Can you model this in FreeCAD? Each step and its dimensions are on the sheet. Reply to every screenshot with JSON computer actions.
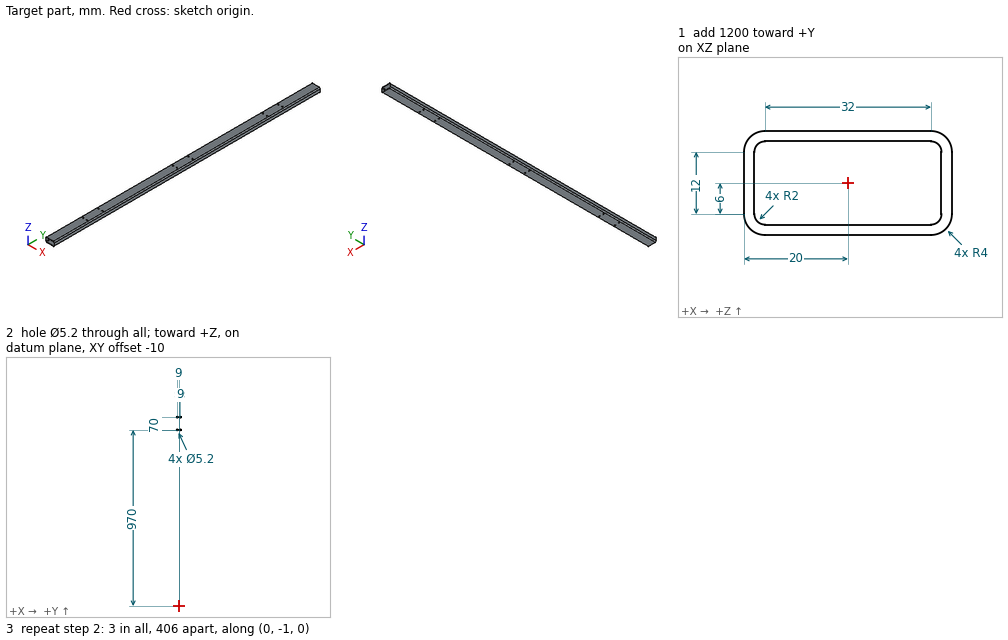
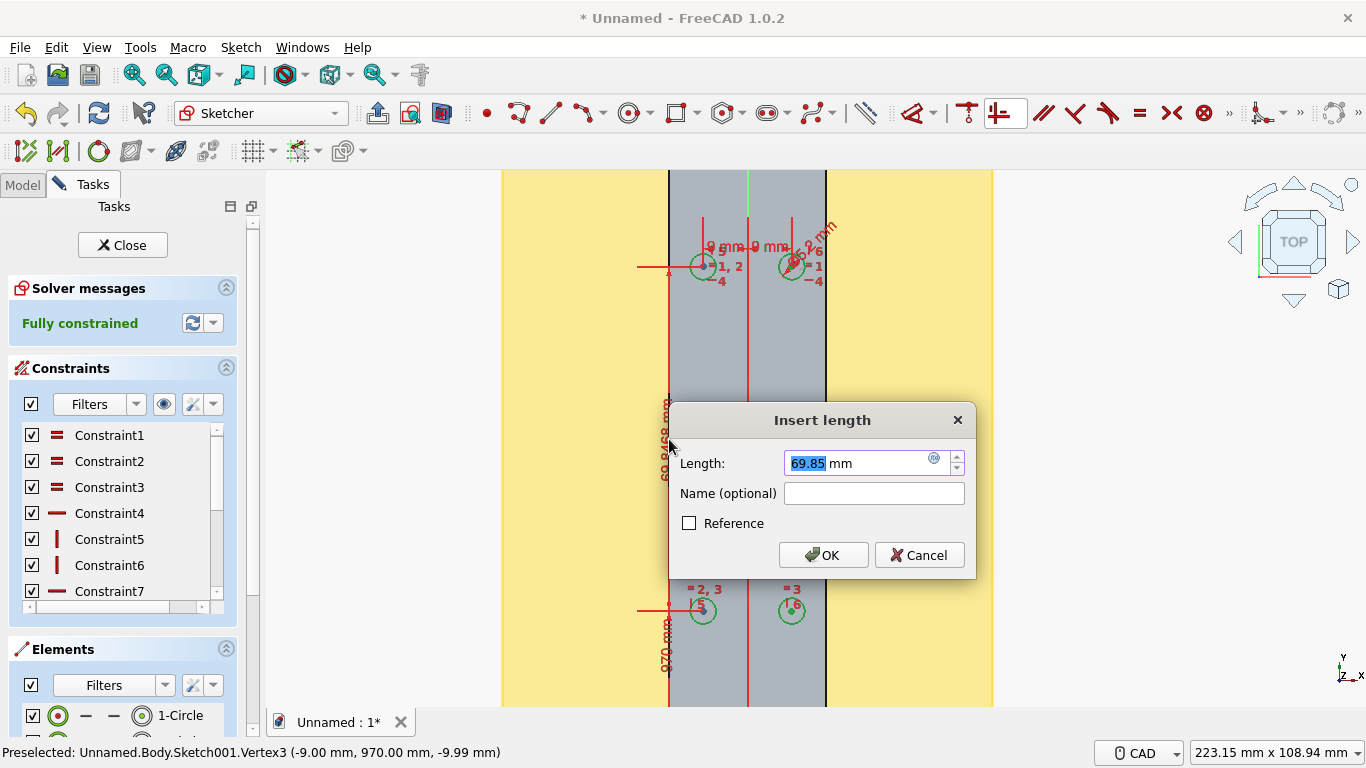
{"action": "type", "text": "70"}
{"action": "key", "text": "Return"}
{"action": "key", "text": "Escape"}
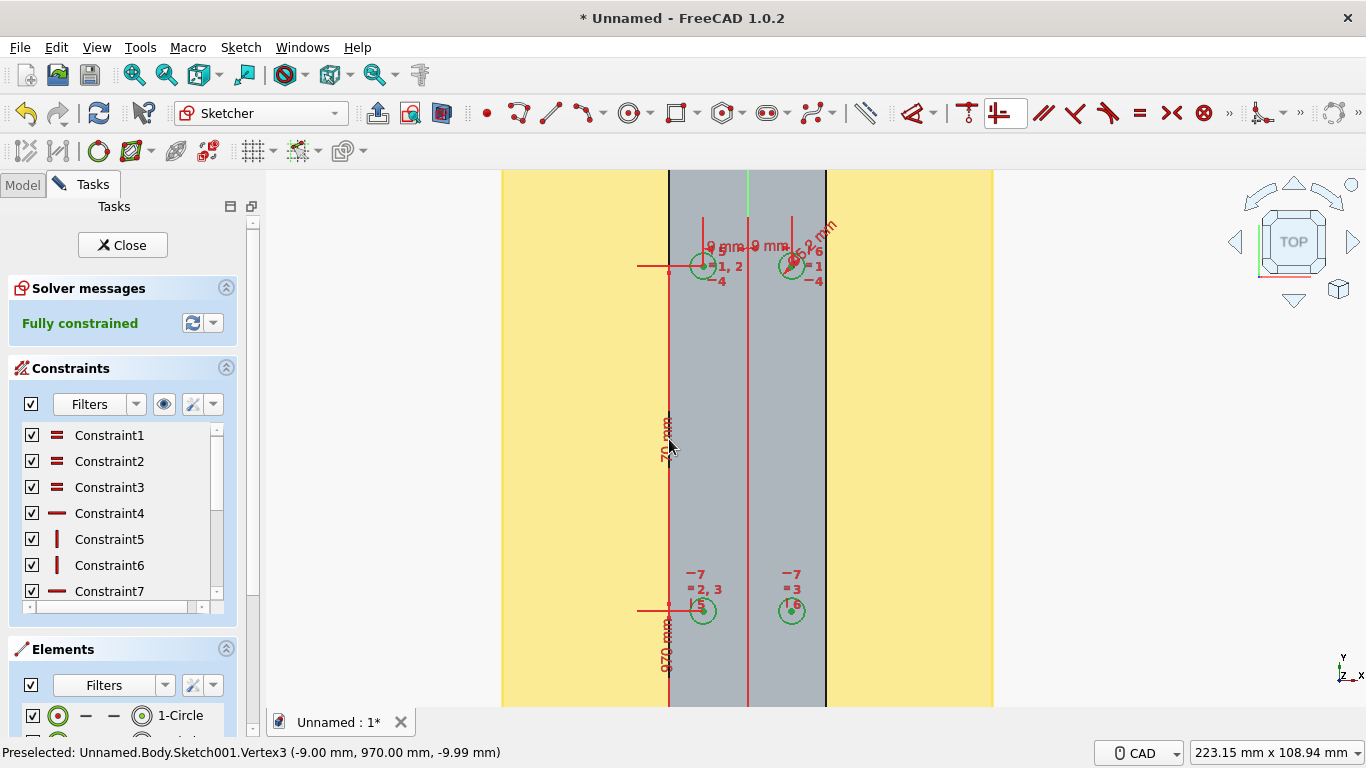
{"action": "left_click", "coordinate": [123, 245]}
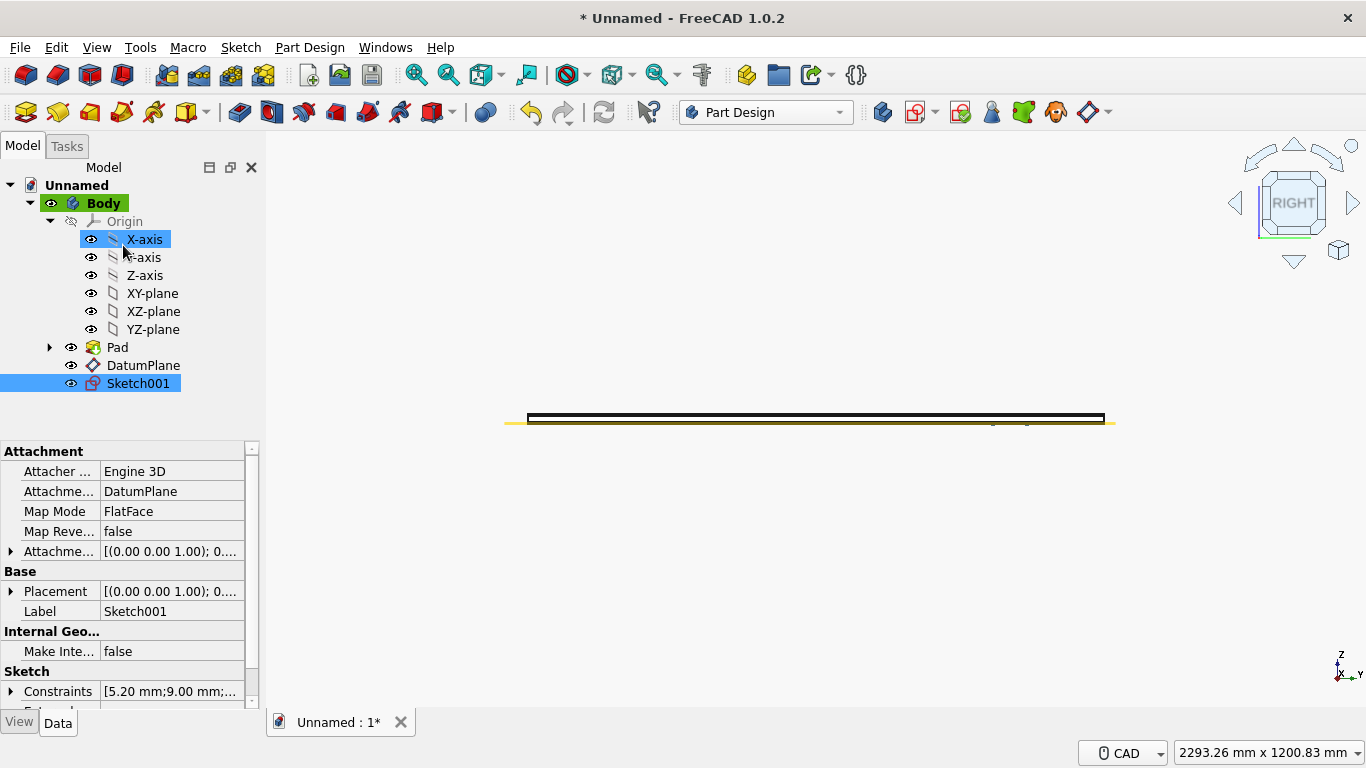
{"action": "left_click", "coordinate": [272, 112]}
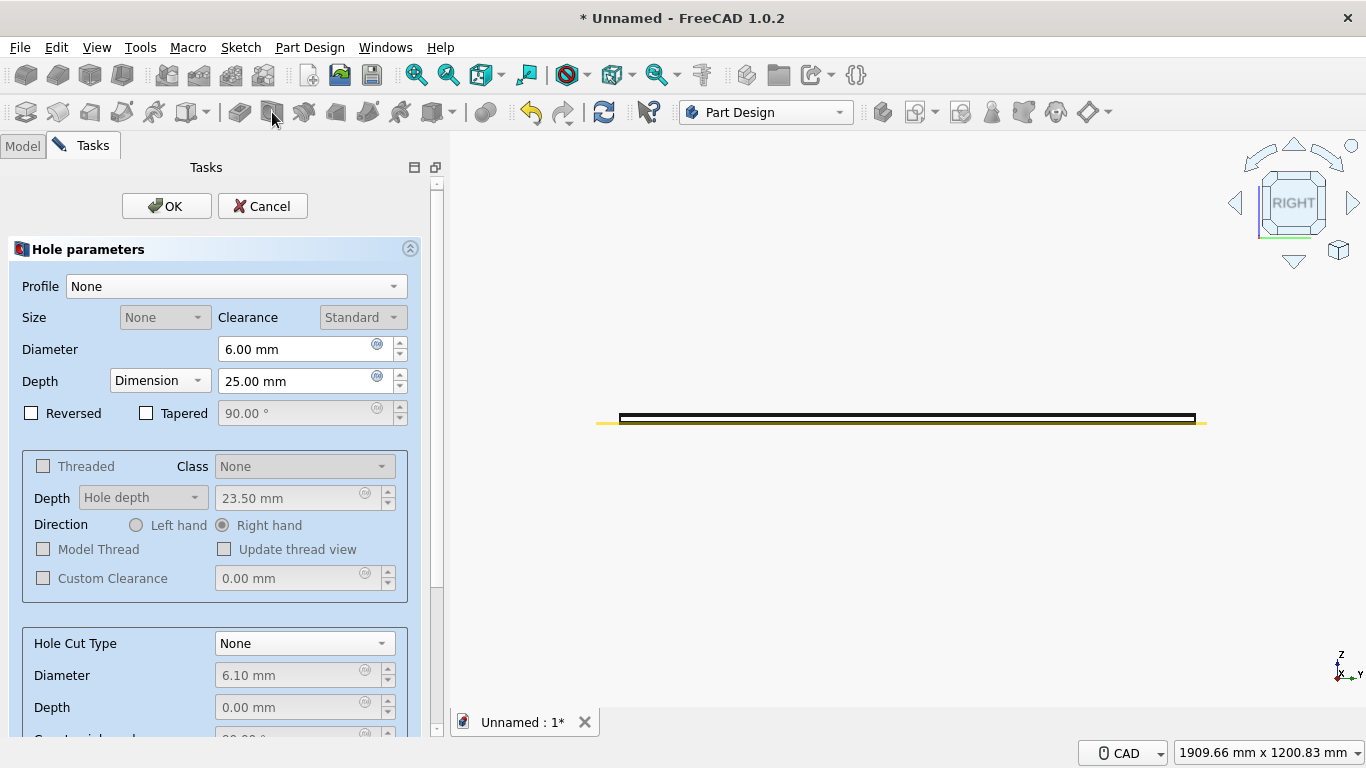
{"action": "triple_click", "coordinate": [305, 349]}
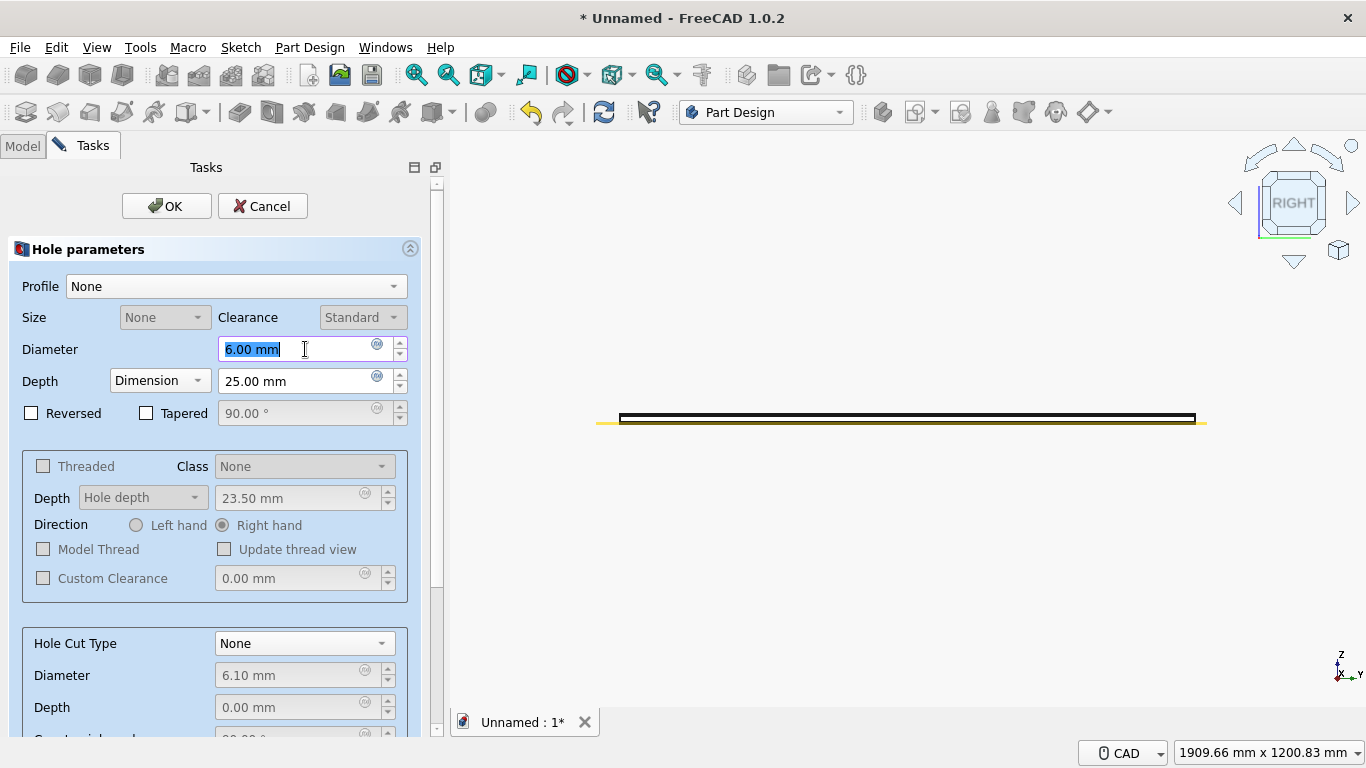
{"action": "type", "text": "5.2"}
{"action": "key", "text": "Tab"}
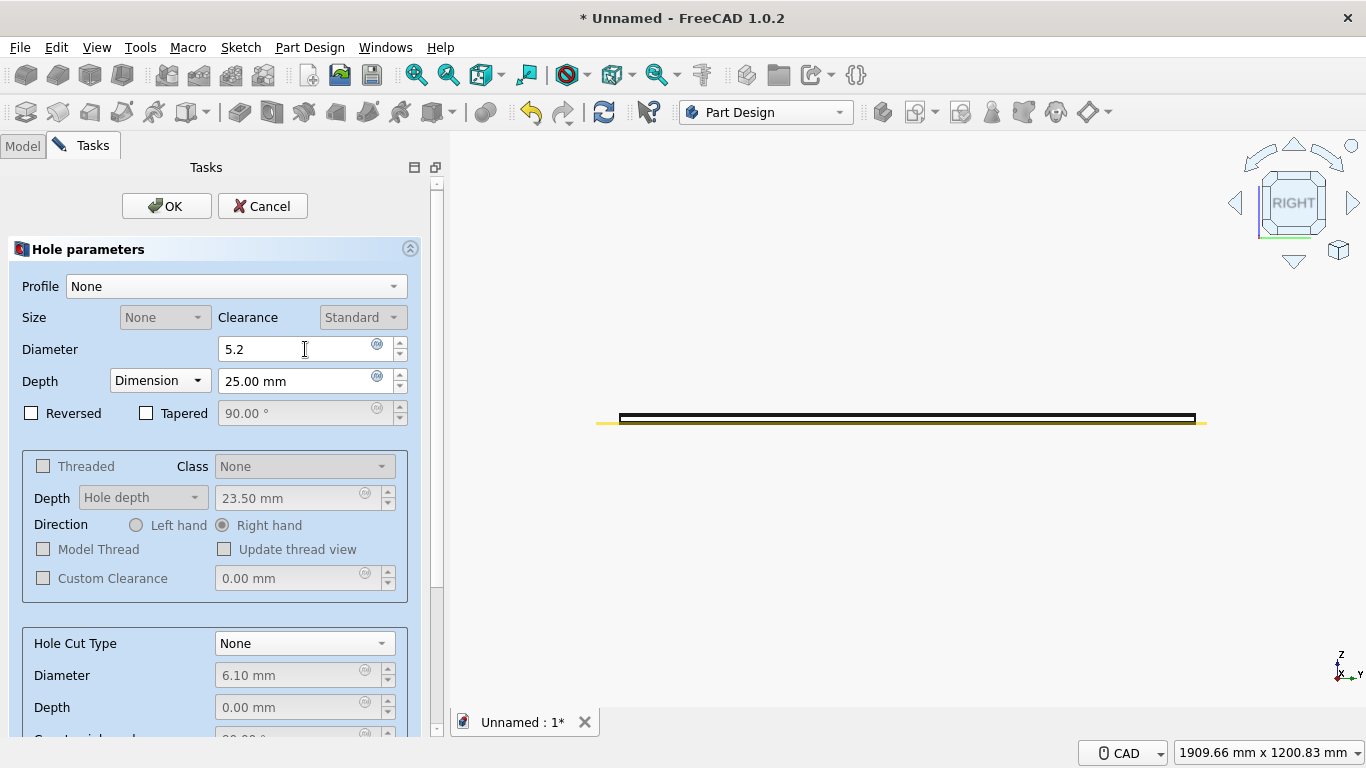
{"action": "left_click", "coordinate": [161, 380]}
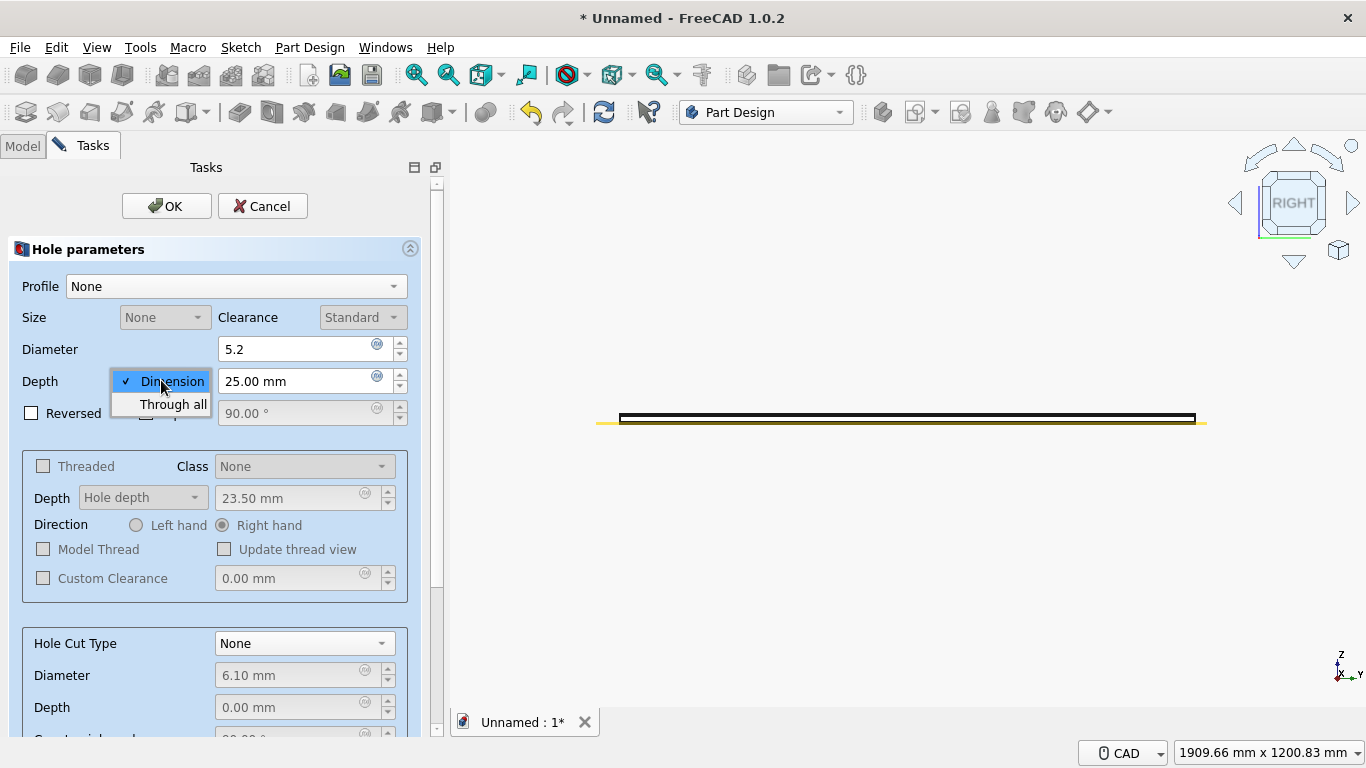
{"action": "left_click", "coordinate": [160, 404]}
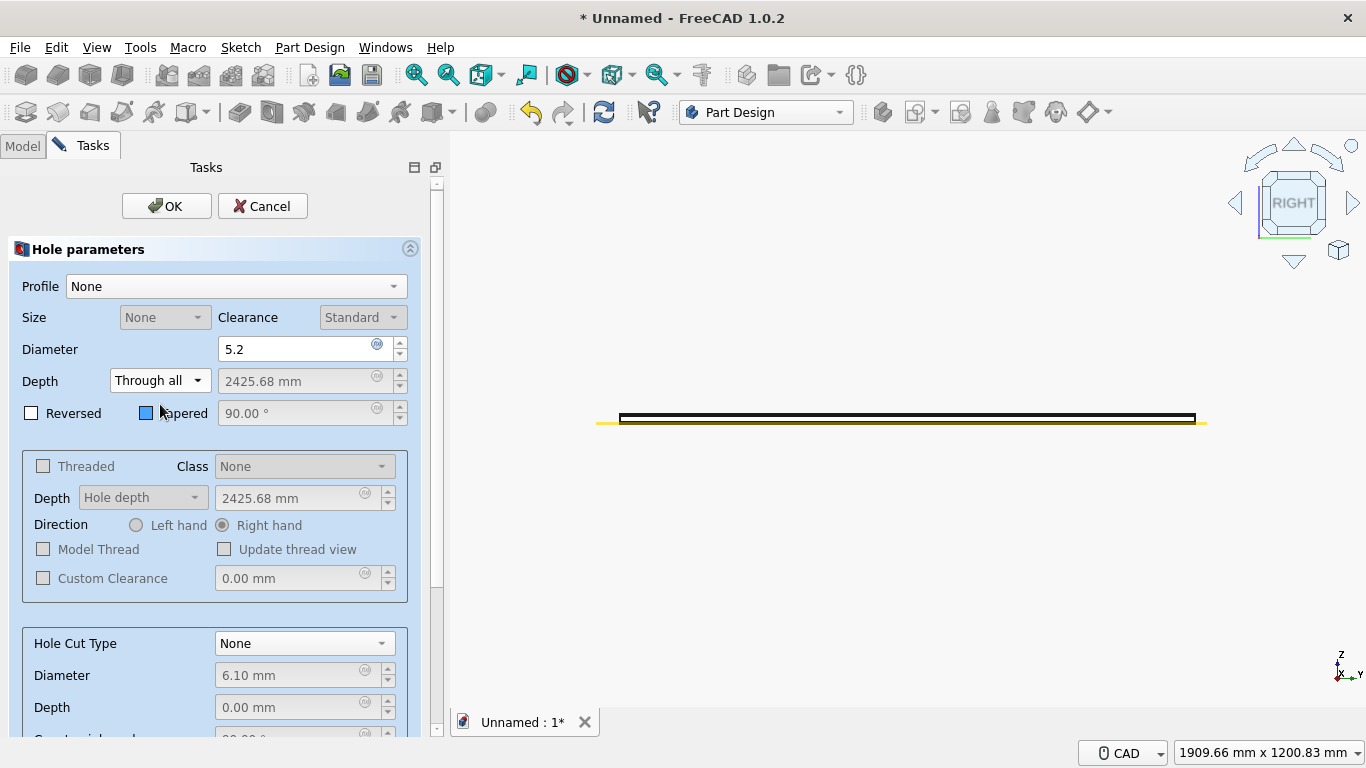
{"action": "left_click", "coordinate": [30, 413]}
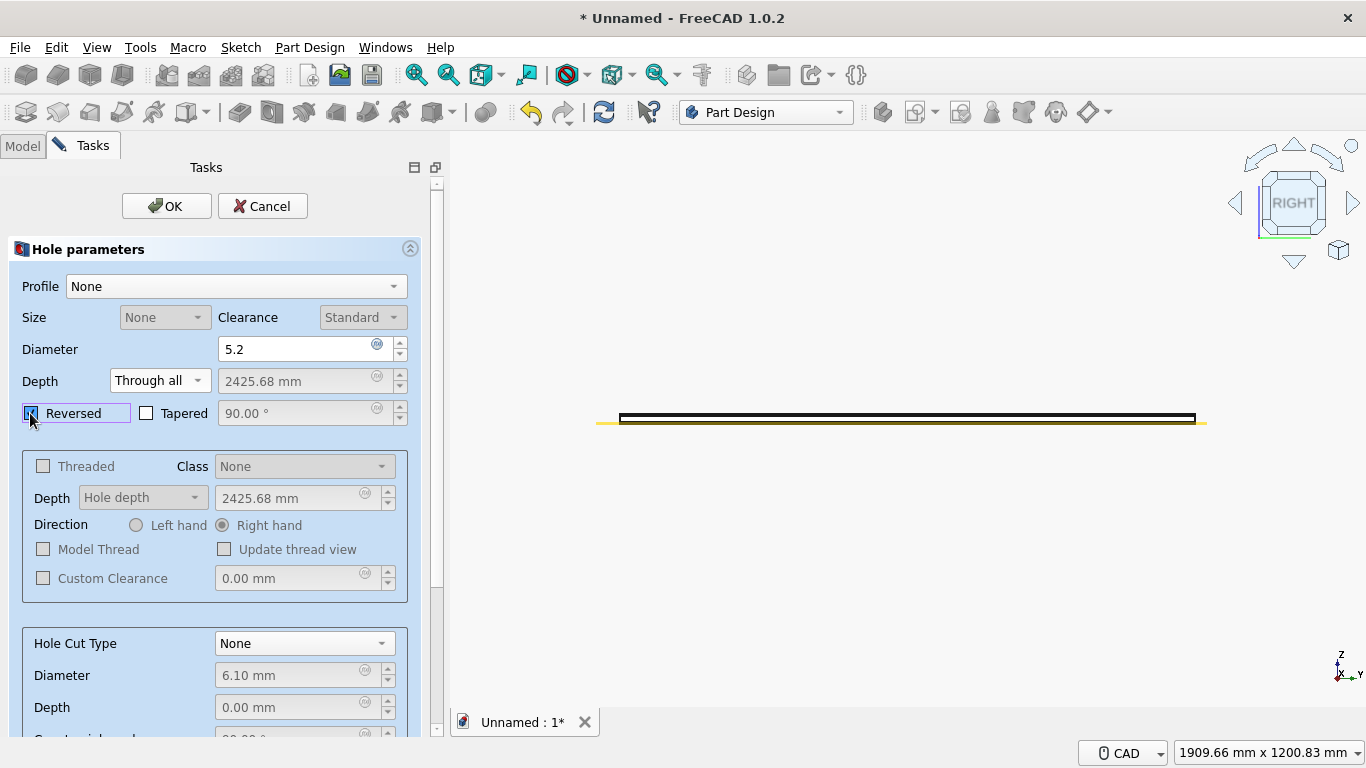
{"action": "left_click", "coordinate": [167, 206]}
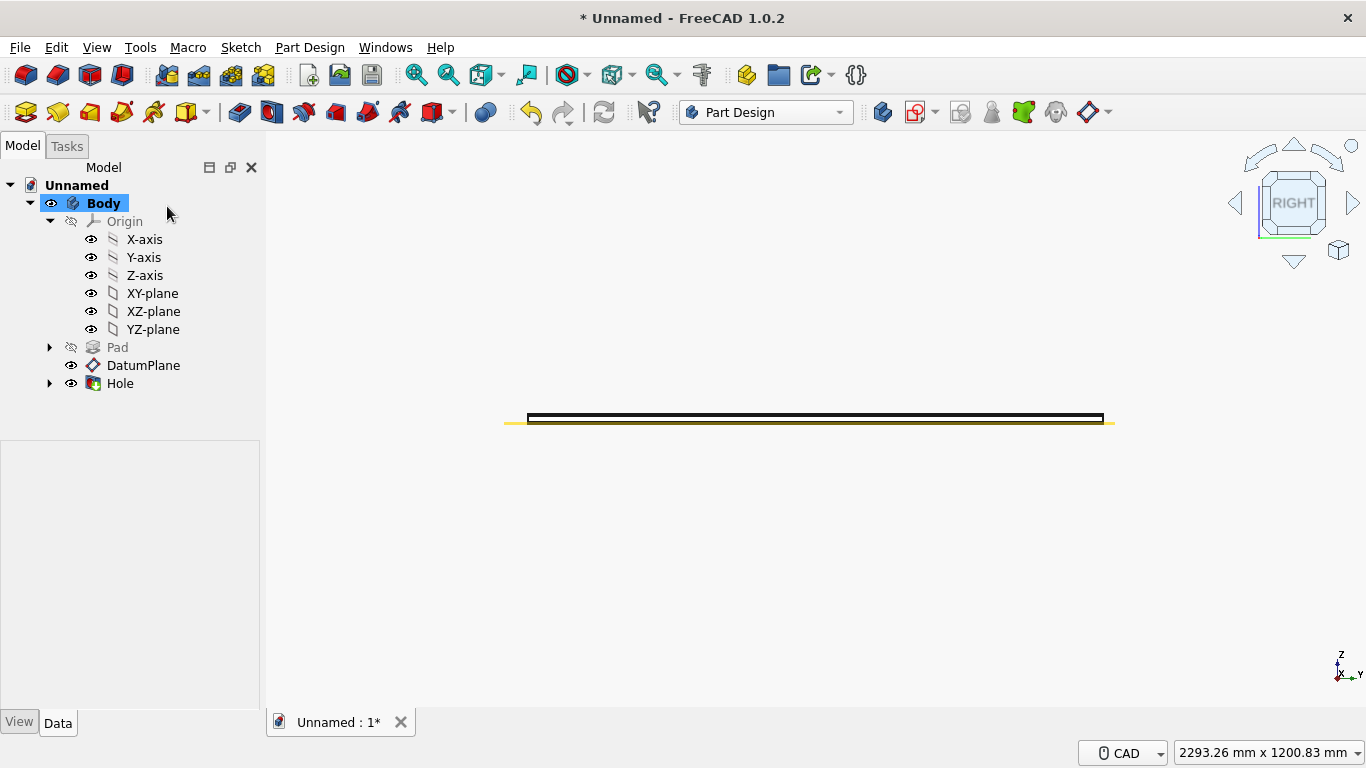
{"action": "left_click", "coordinate": [116, 365]}
{"action": "key", "text": "space"}